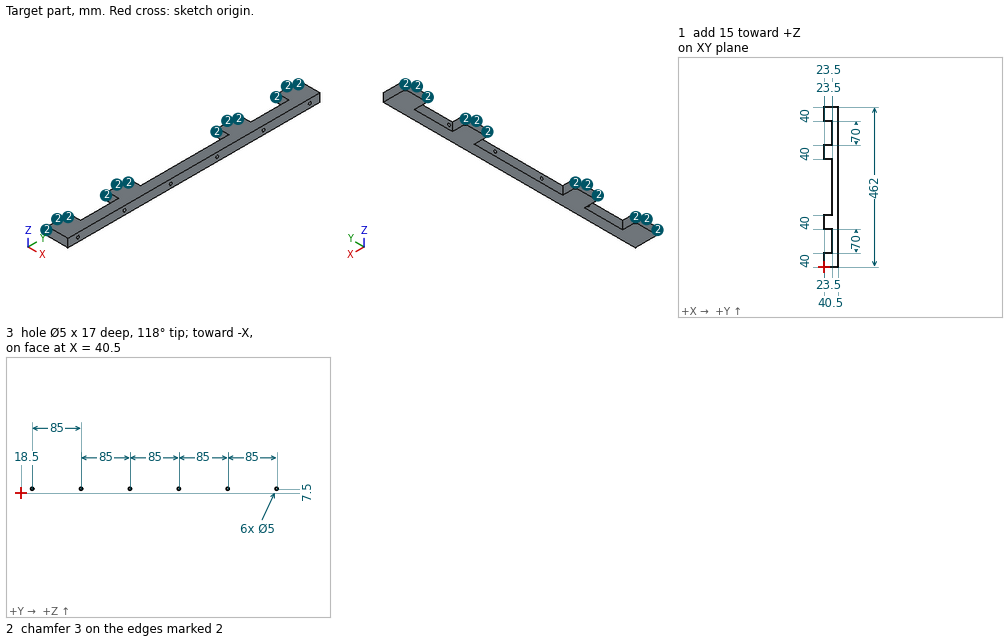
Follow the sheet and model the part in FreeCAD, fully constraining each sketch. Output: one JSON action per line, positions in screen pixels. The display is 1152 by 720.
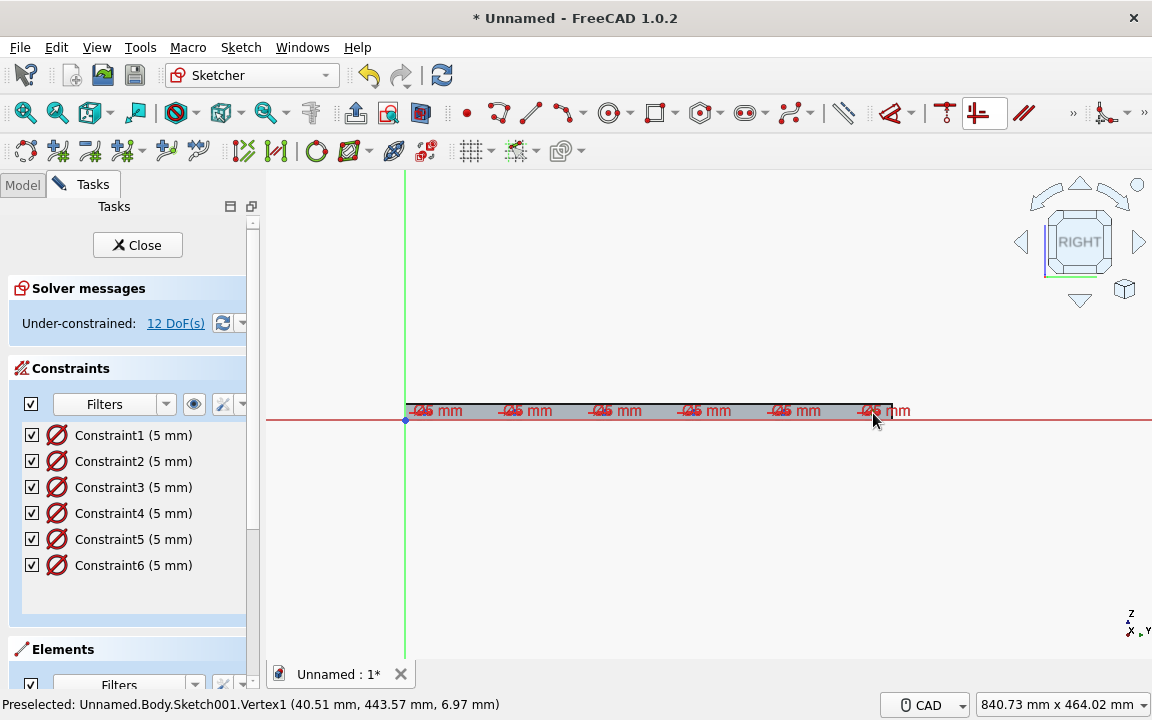
{"action": "left_click", "coordinate": [783, 413]}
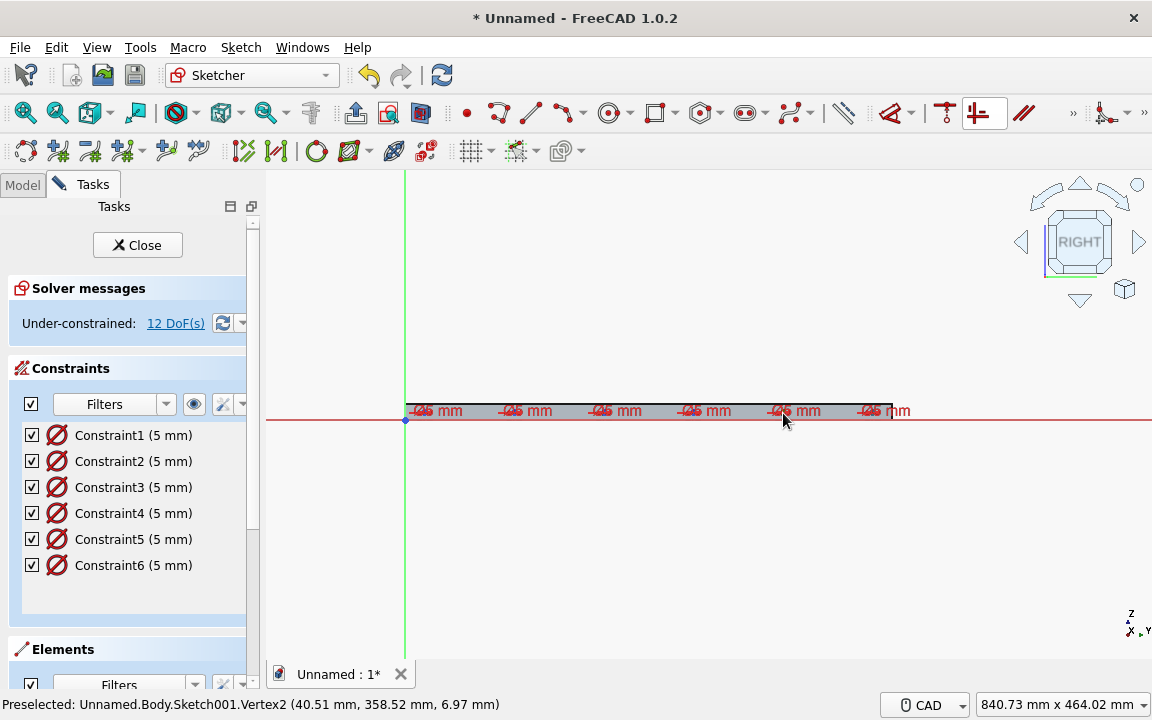
{"action": "key", "text": "h"}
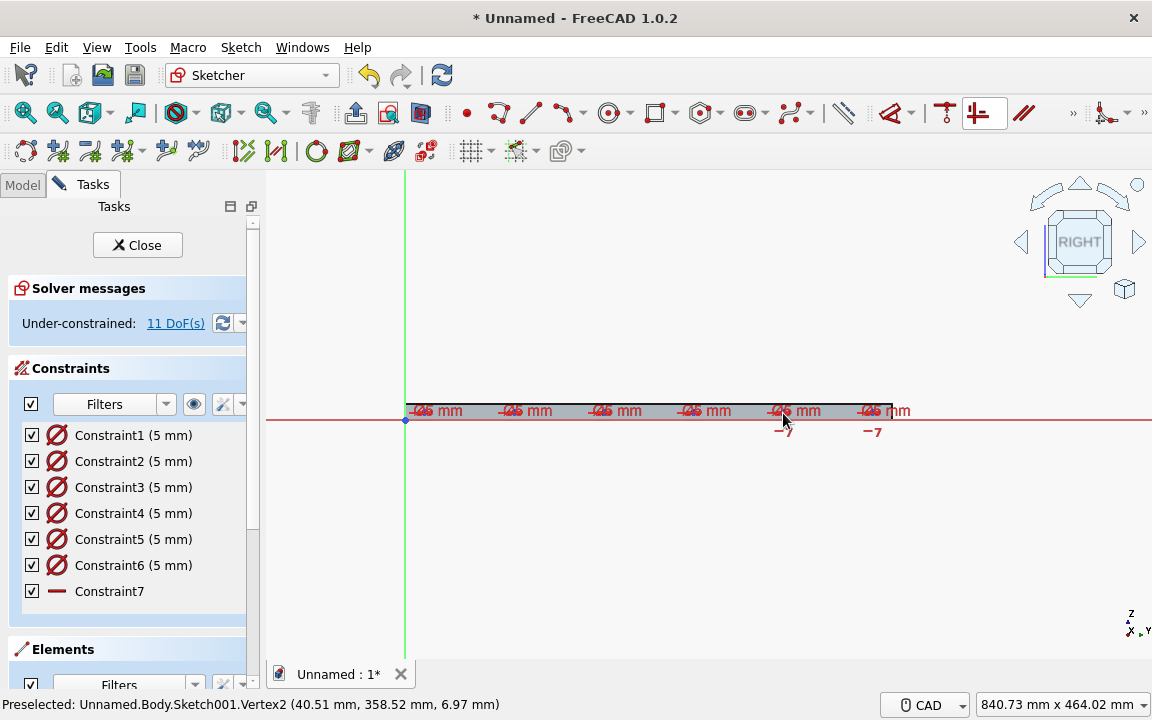
{"action": "left_click", "coordinate": [783, 413]}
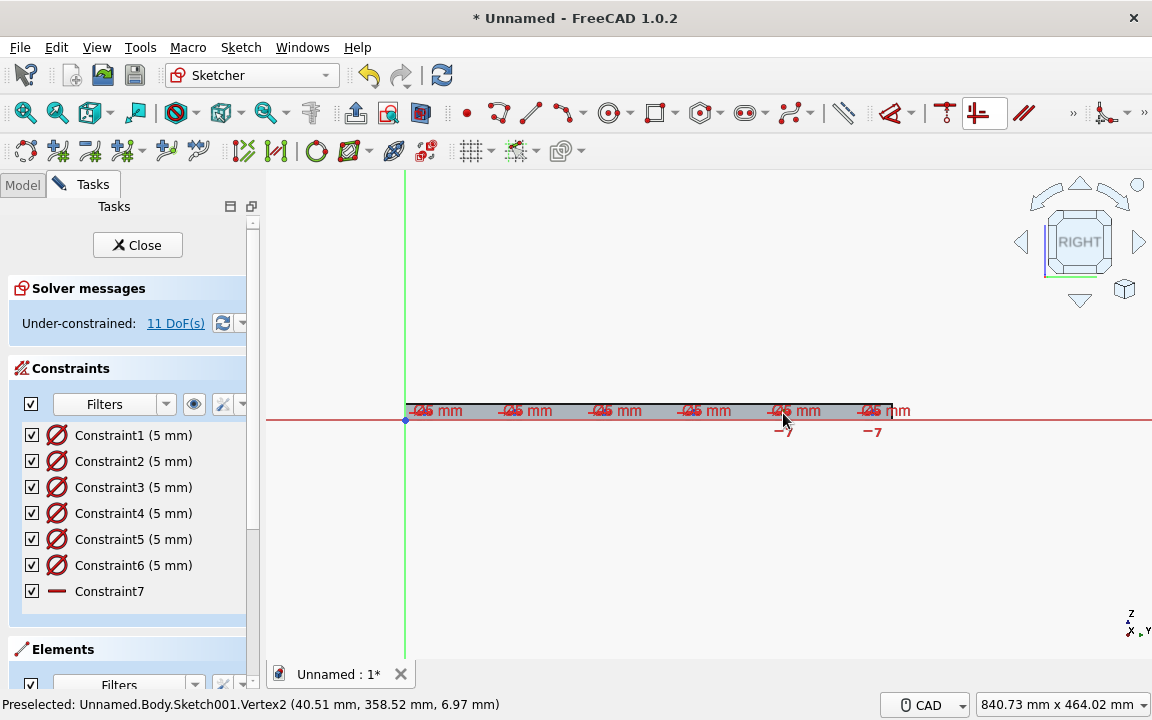
{"action": "left_click", "coordinate": [694, 413]}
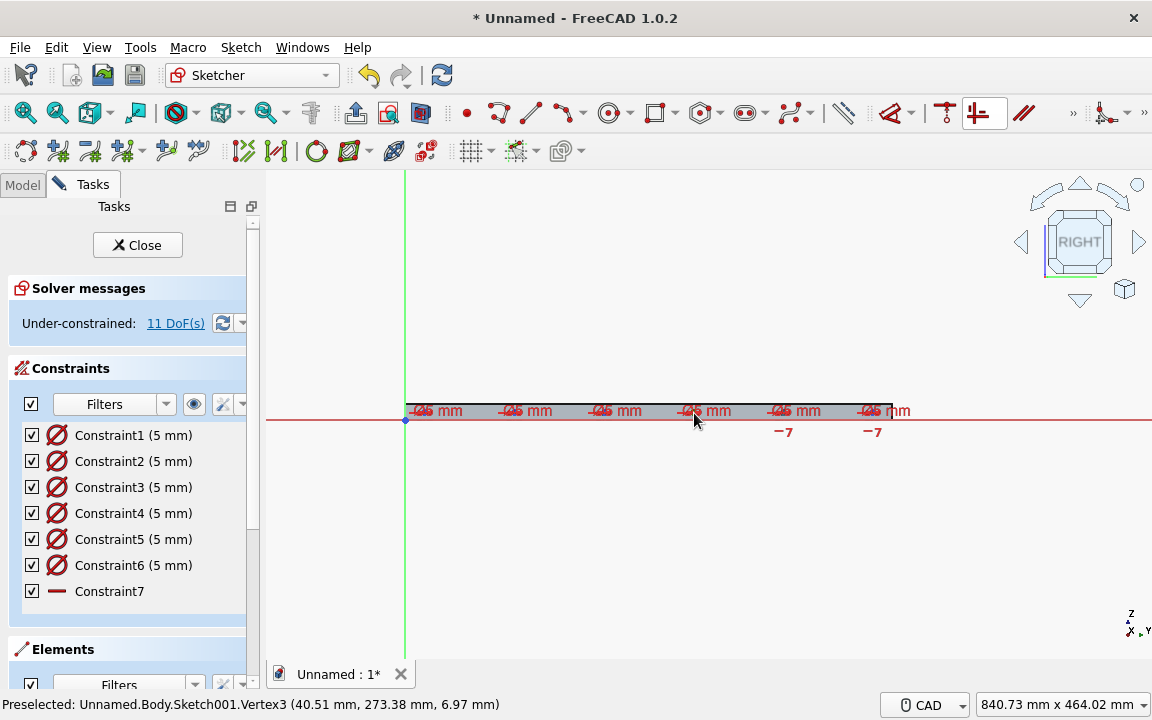
{"action": "key", "text": "h"}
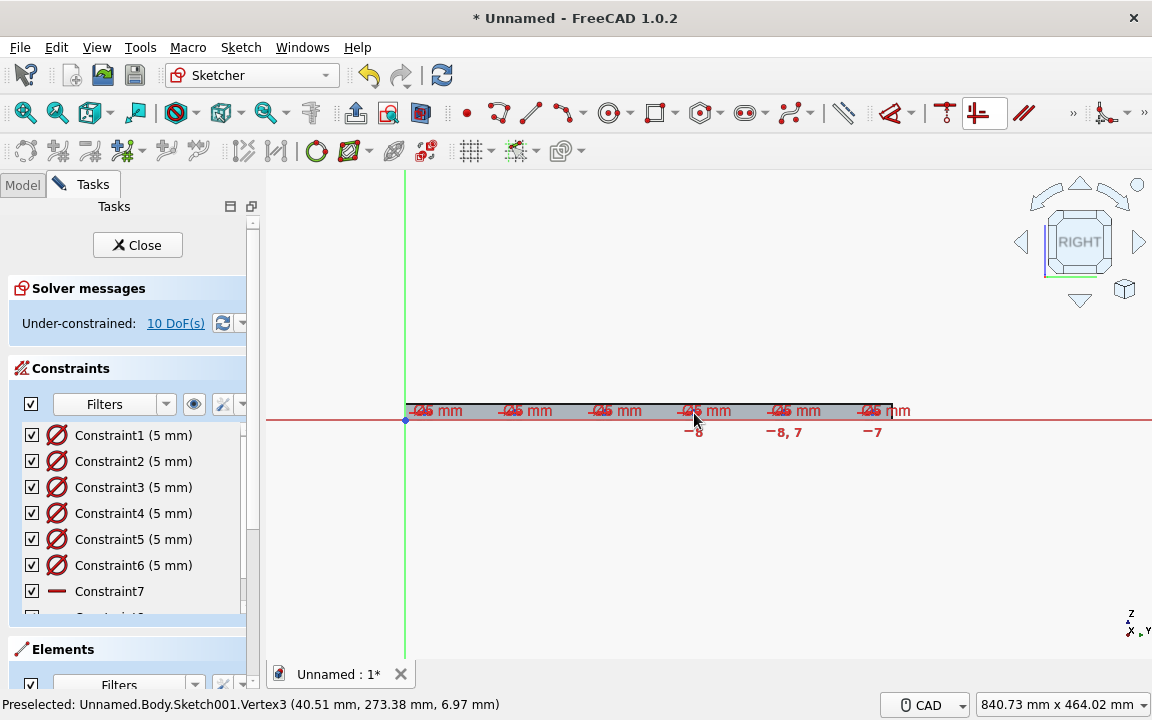
{"action": "left_click", "coordinate": [694, 413]}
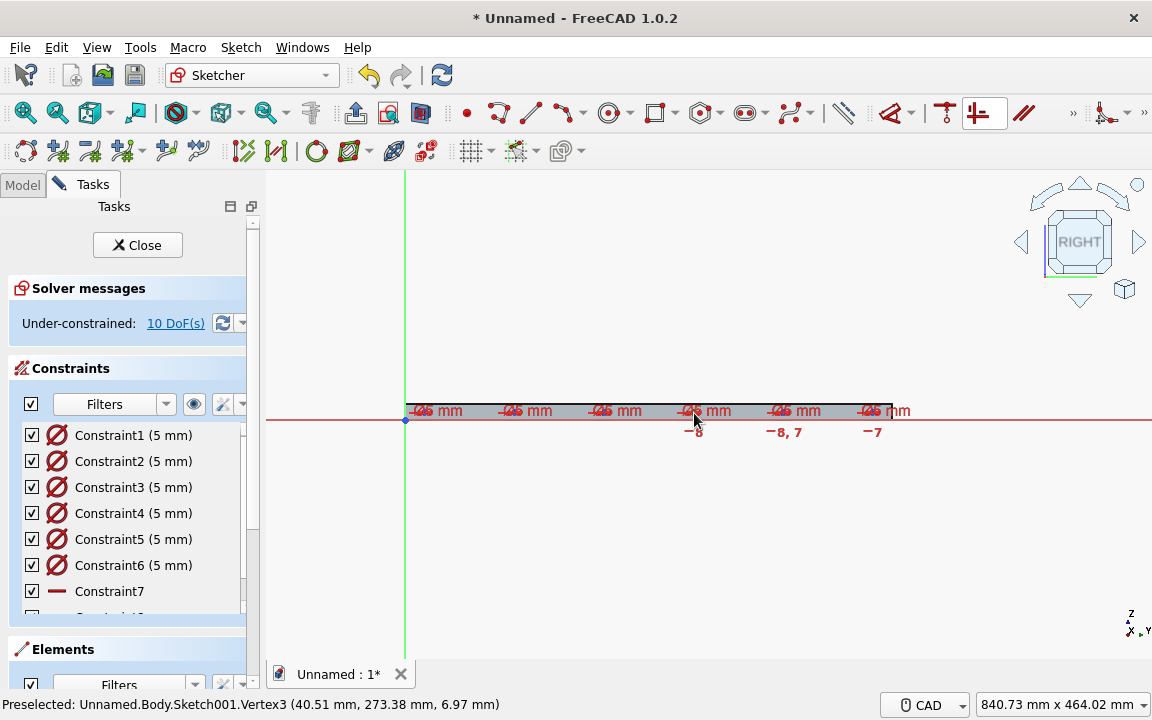
{"action": "left_click", "coordinate": [604, 413]}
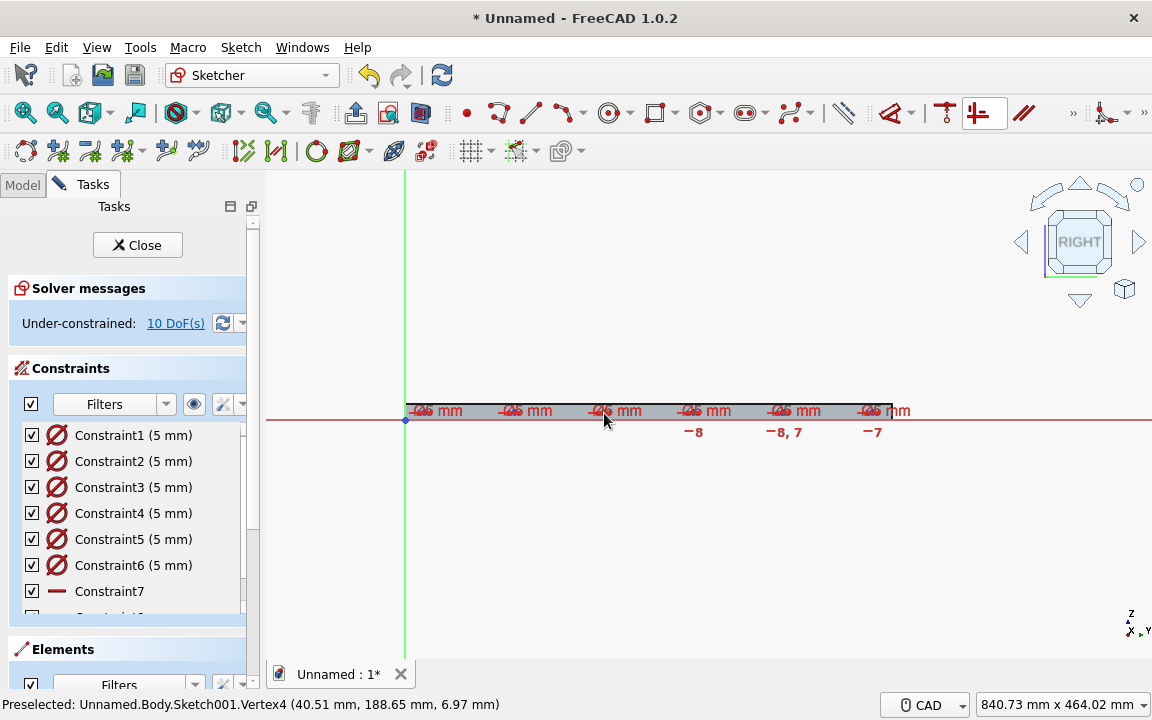
{"action": "key", "text": "h"}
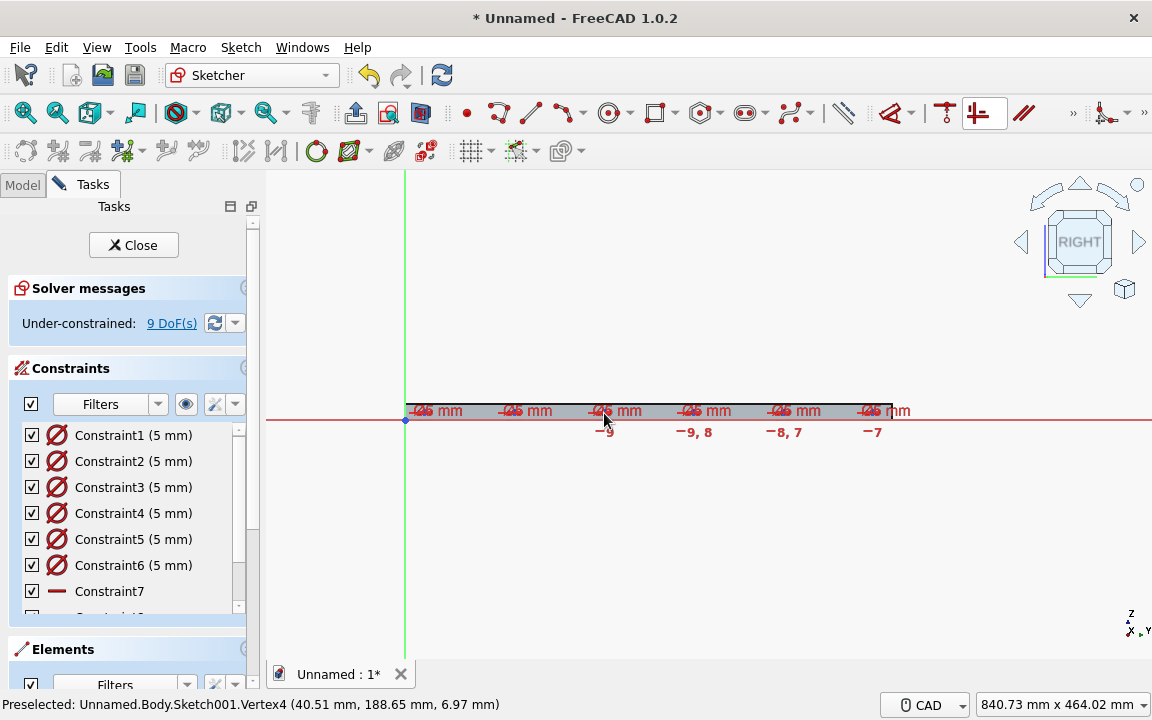
{"action": "left_click", "coordinate": [604, 413]}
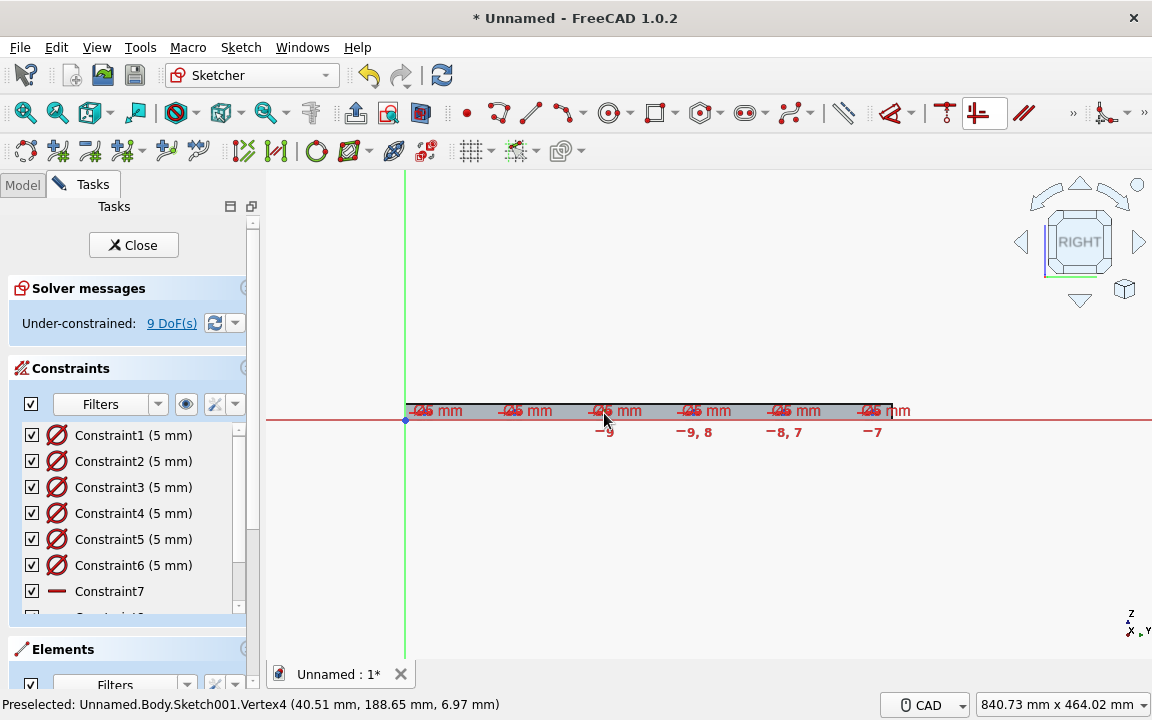
{"action": "left_click", "coordinate": [515, 413]}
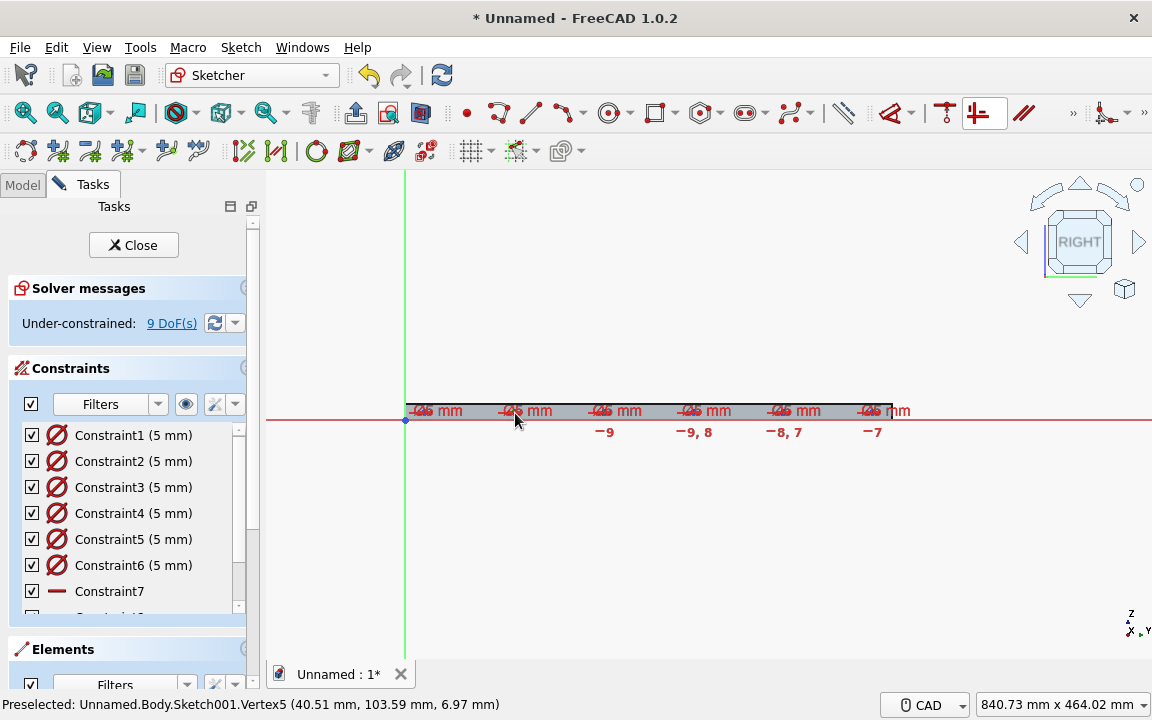
{"action": "key", "text": "h"}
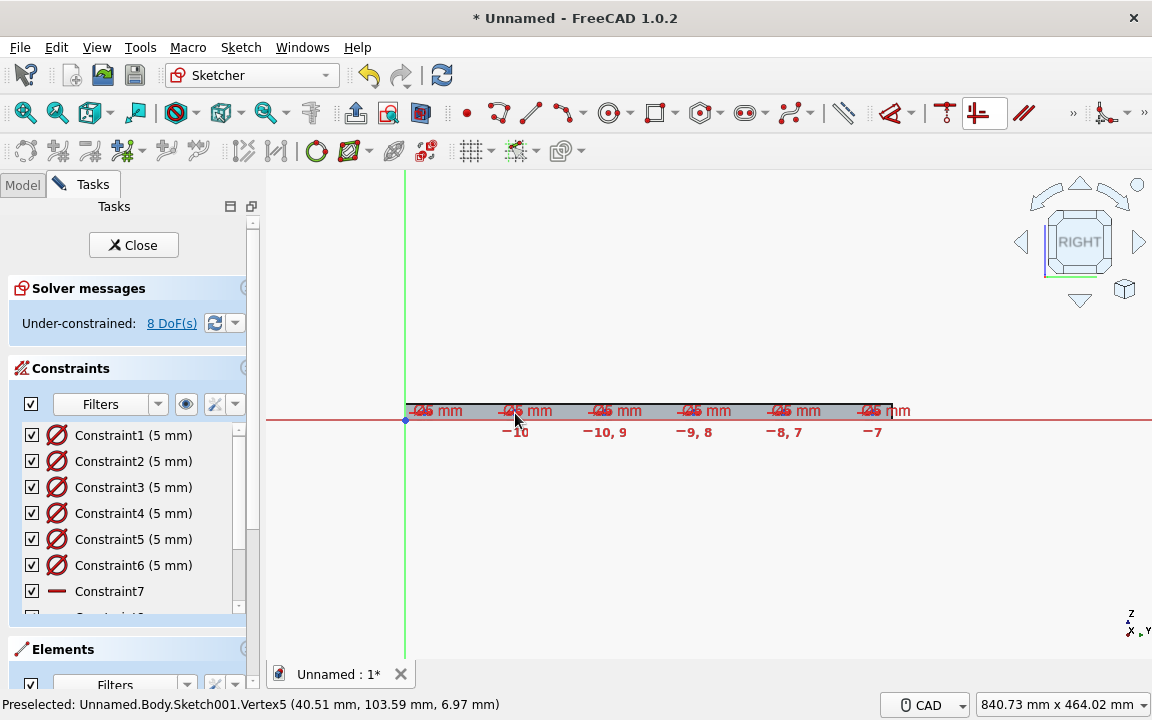
{"action": "left_click", "coordinate": [515, 413]}